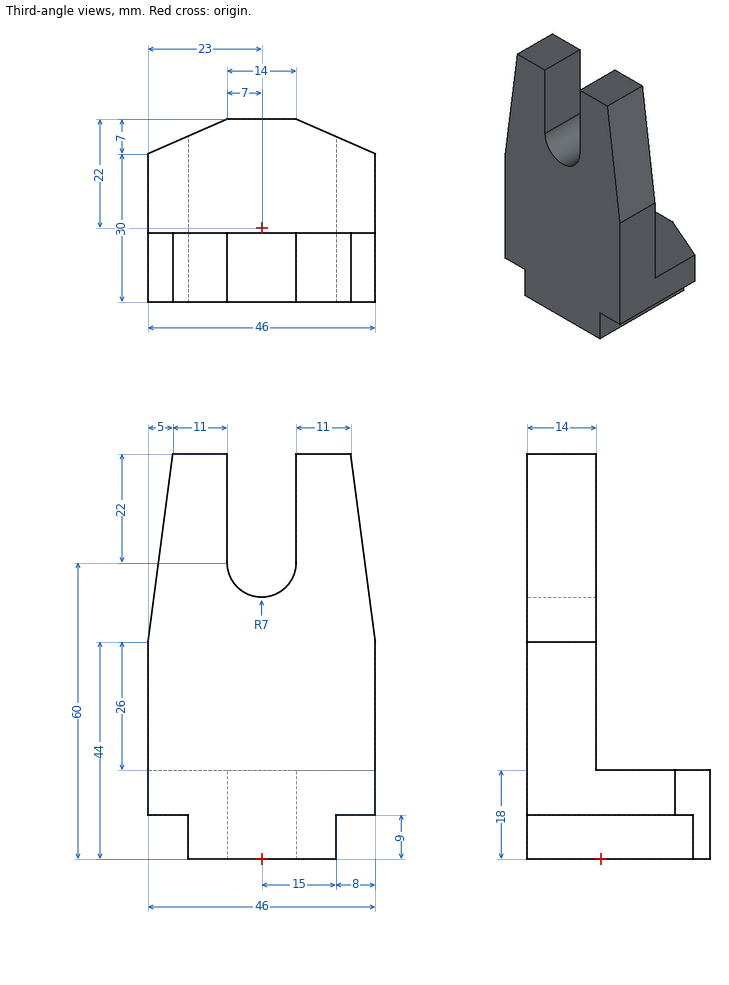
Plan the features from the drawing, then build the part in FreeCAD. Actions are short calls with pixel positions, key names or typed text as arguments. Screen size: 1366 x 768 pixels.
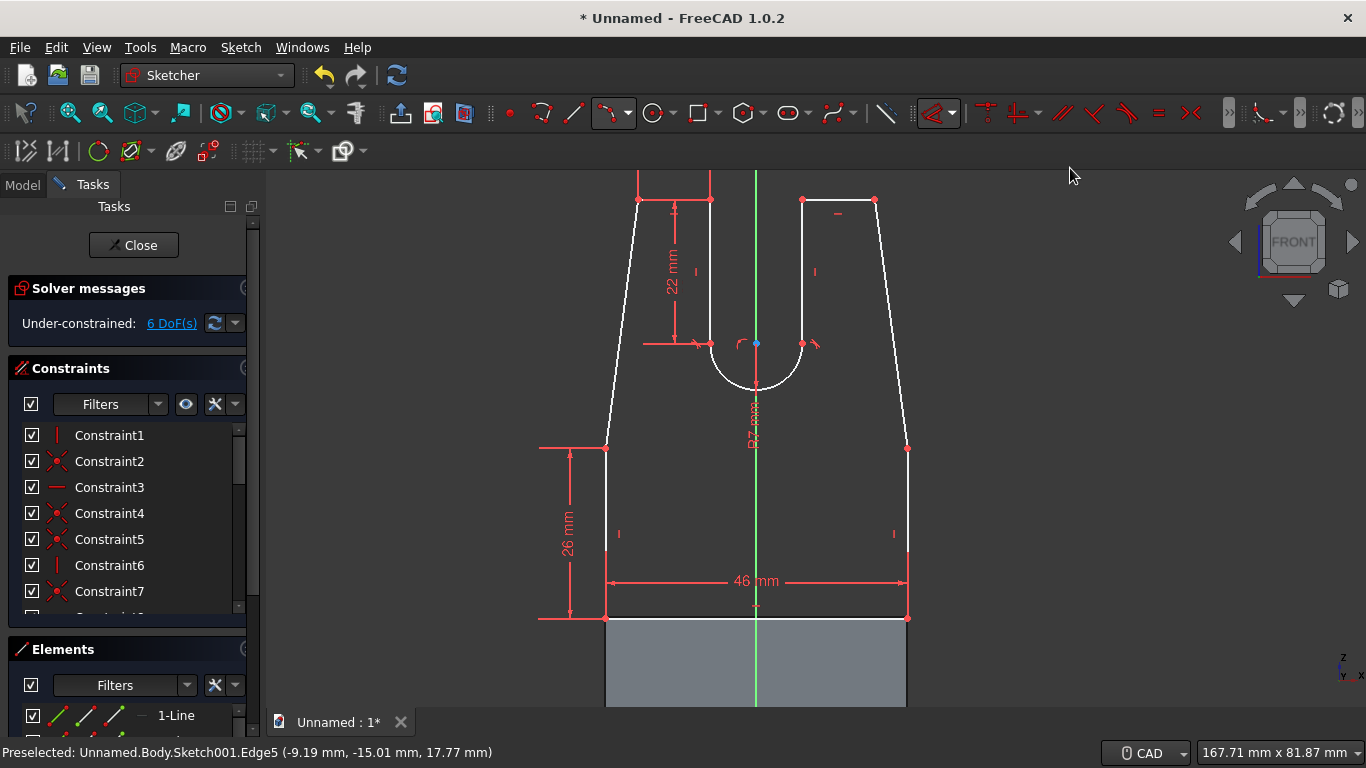
click(908, 568)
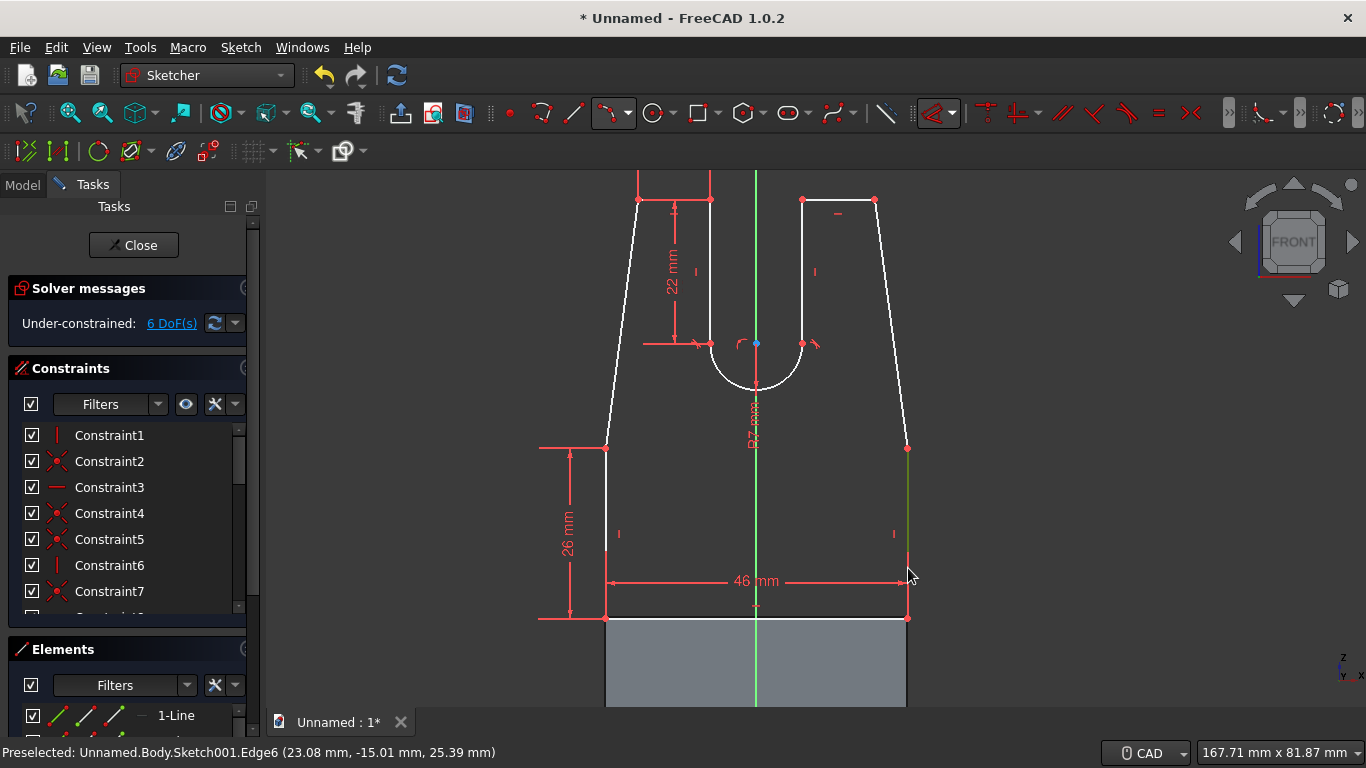
click(954, 114)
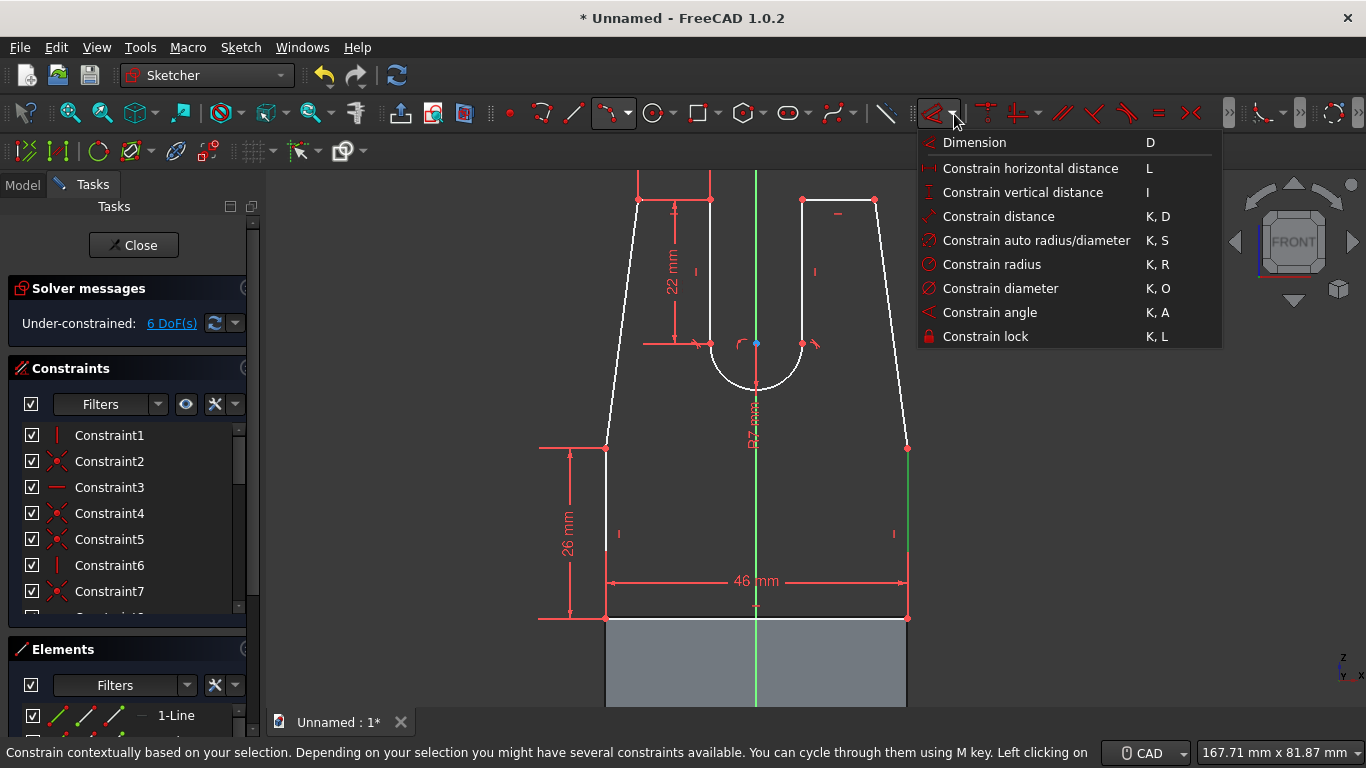
click(1070, 192)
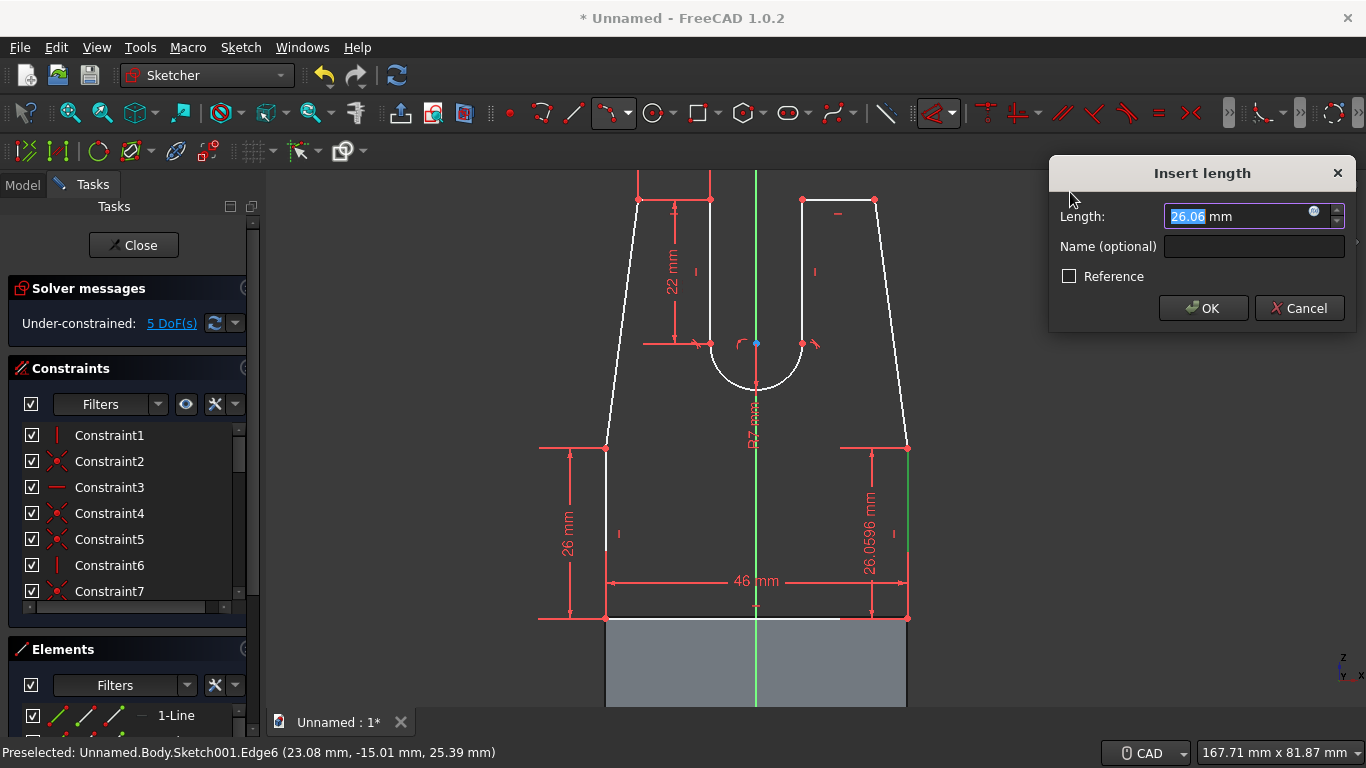
text(26)
key(Return)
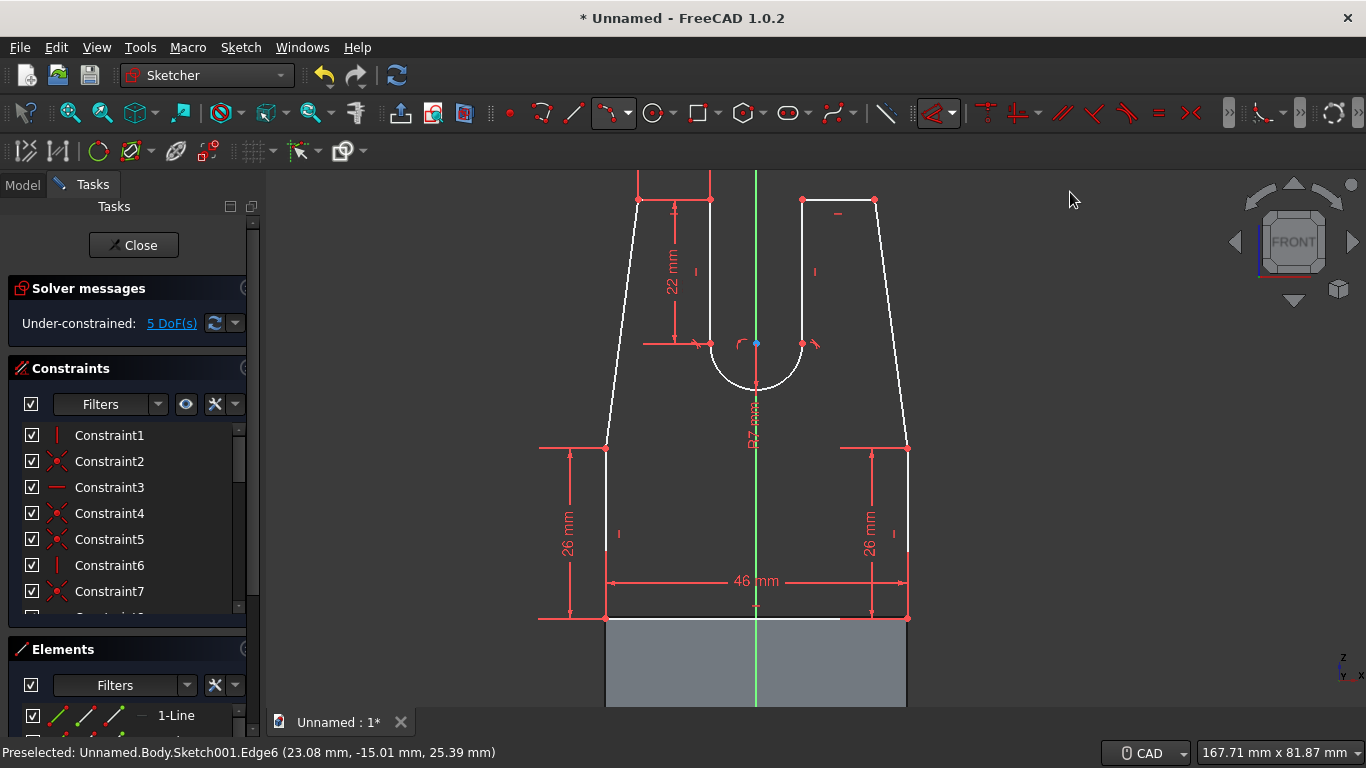
click(853, 200)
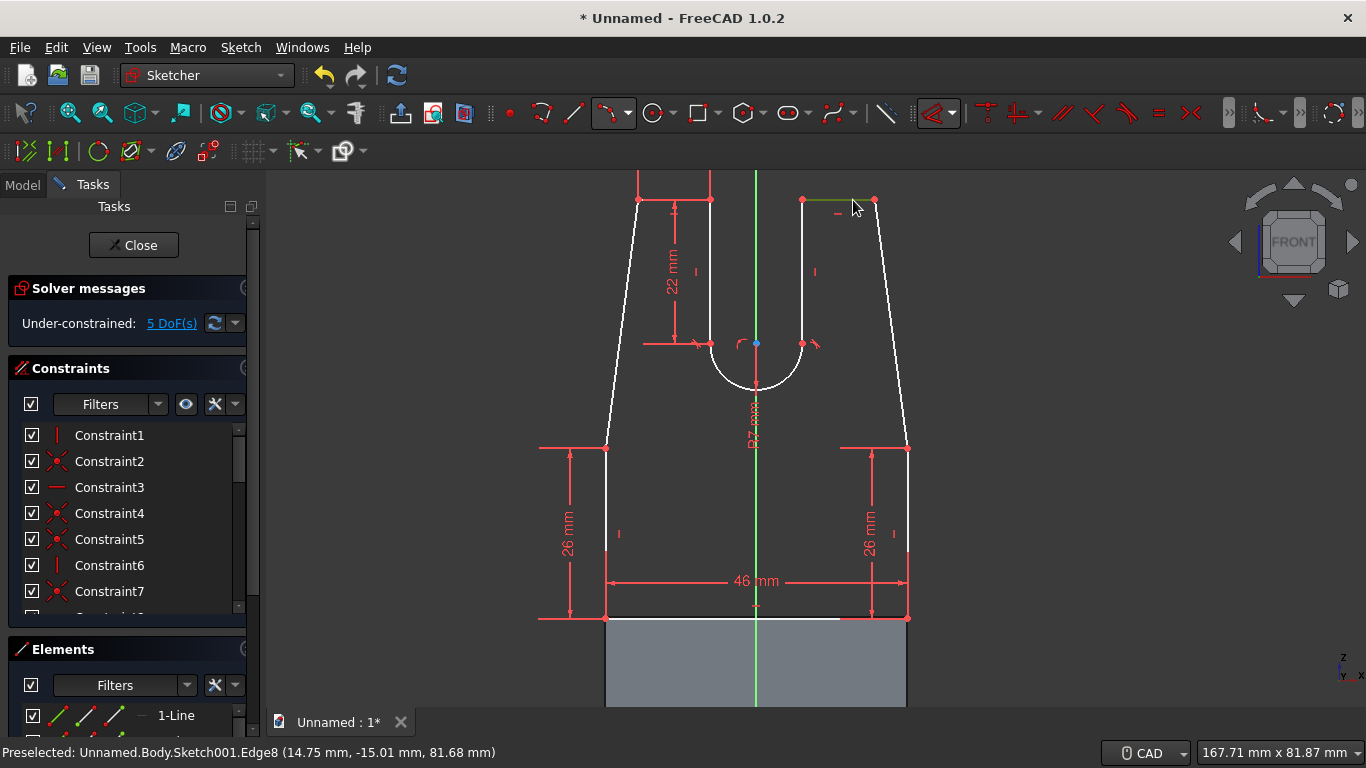
click(954, 114)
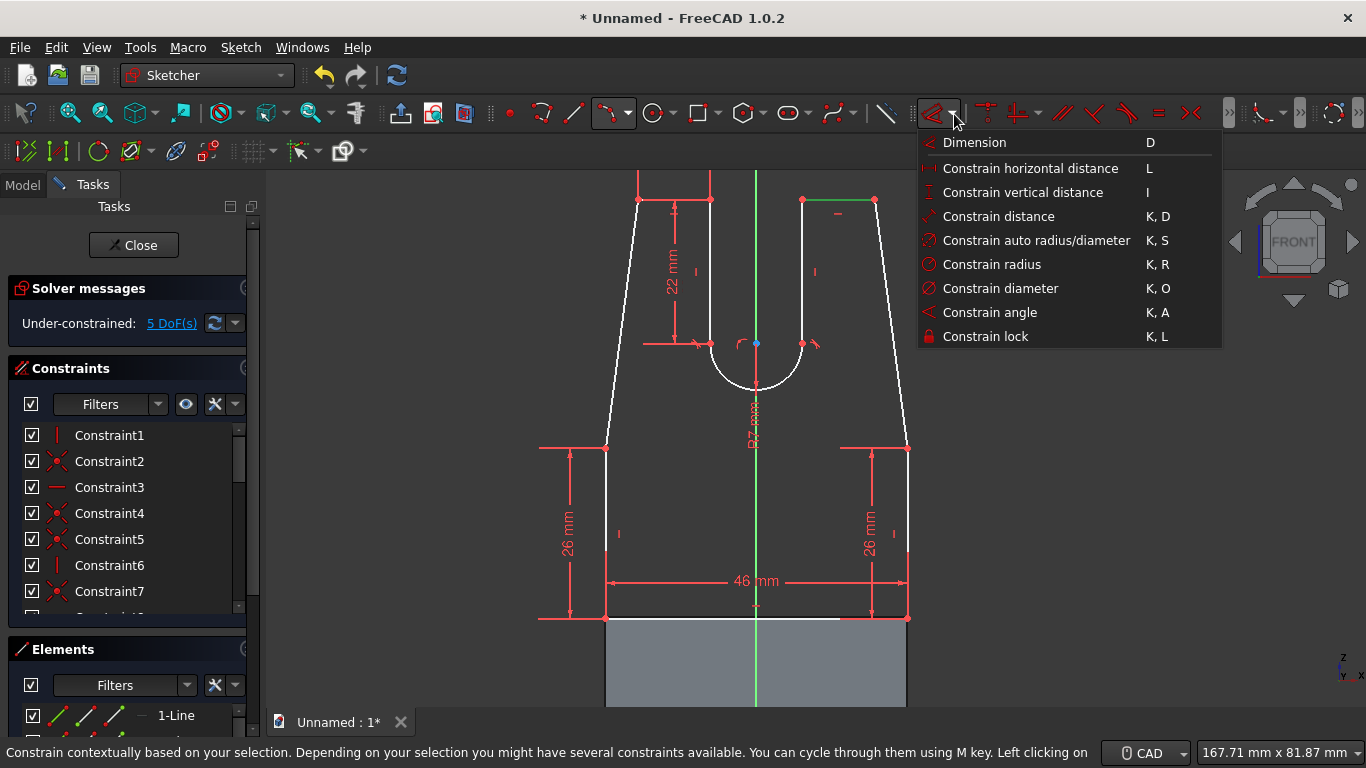
click(1070, 168)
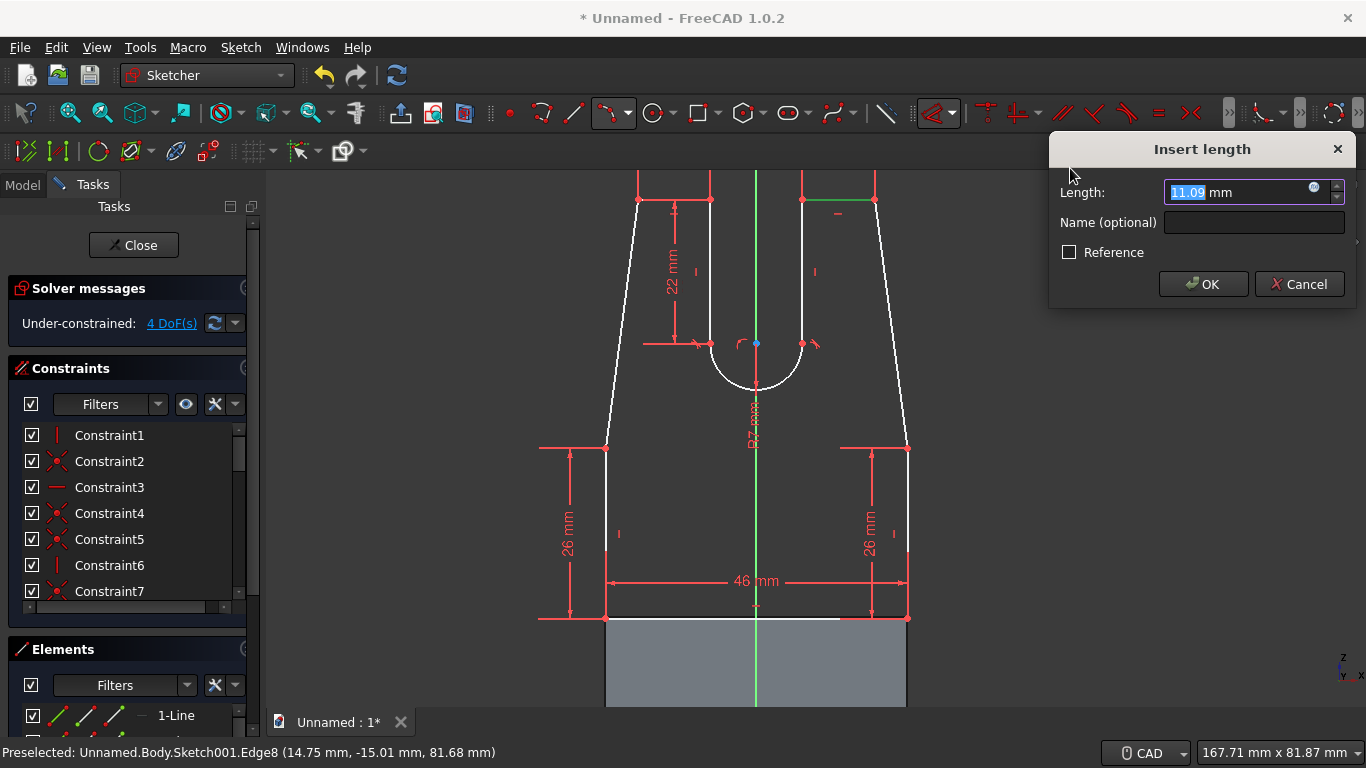
text(11)
key(Return)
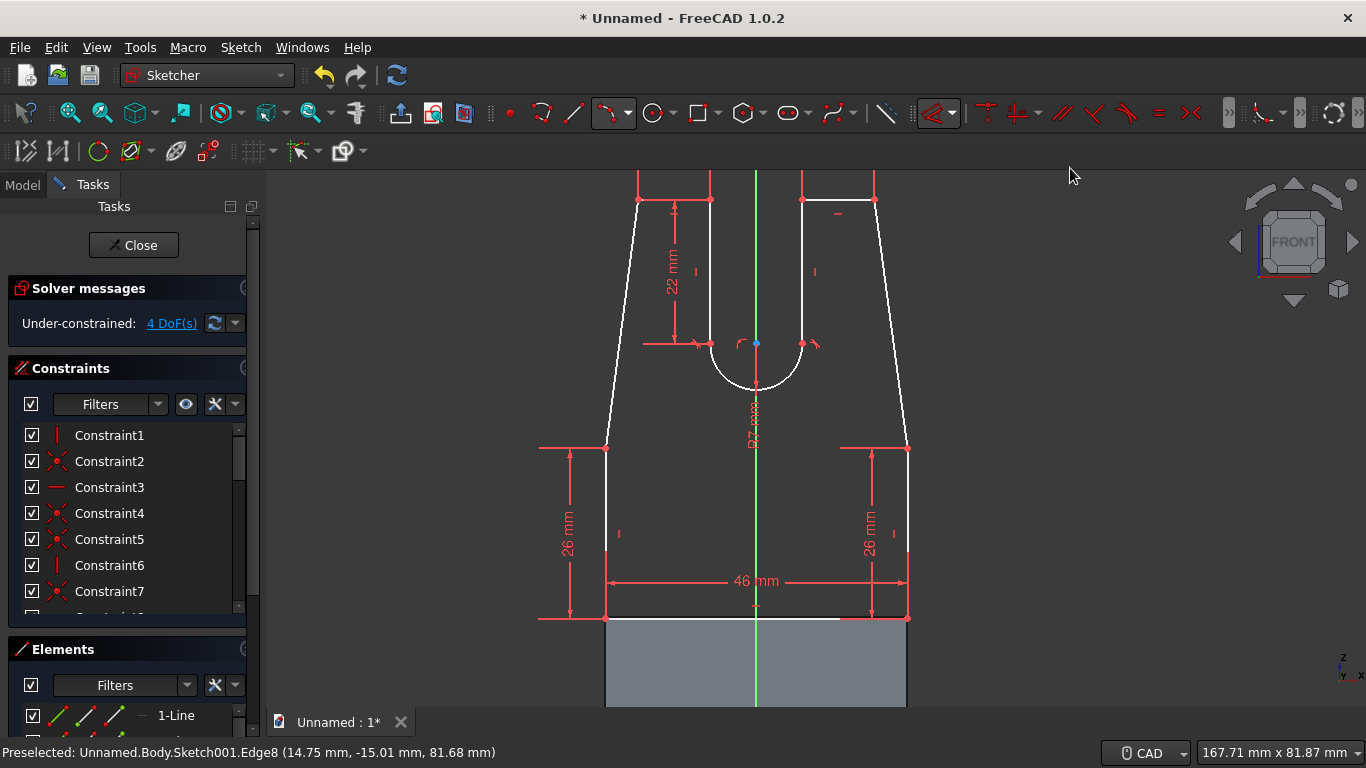
click(802, 243)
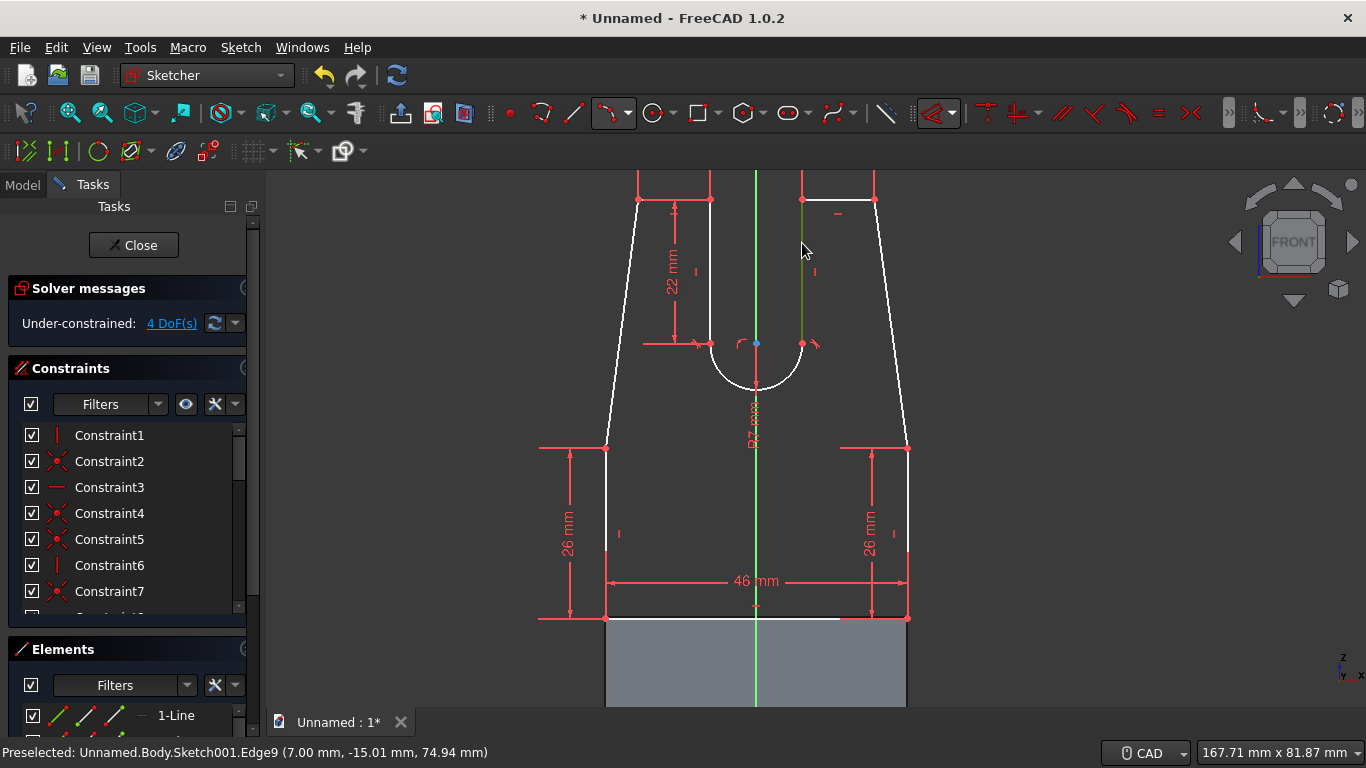
click(954, 114)